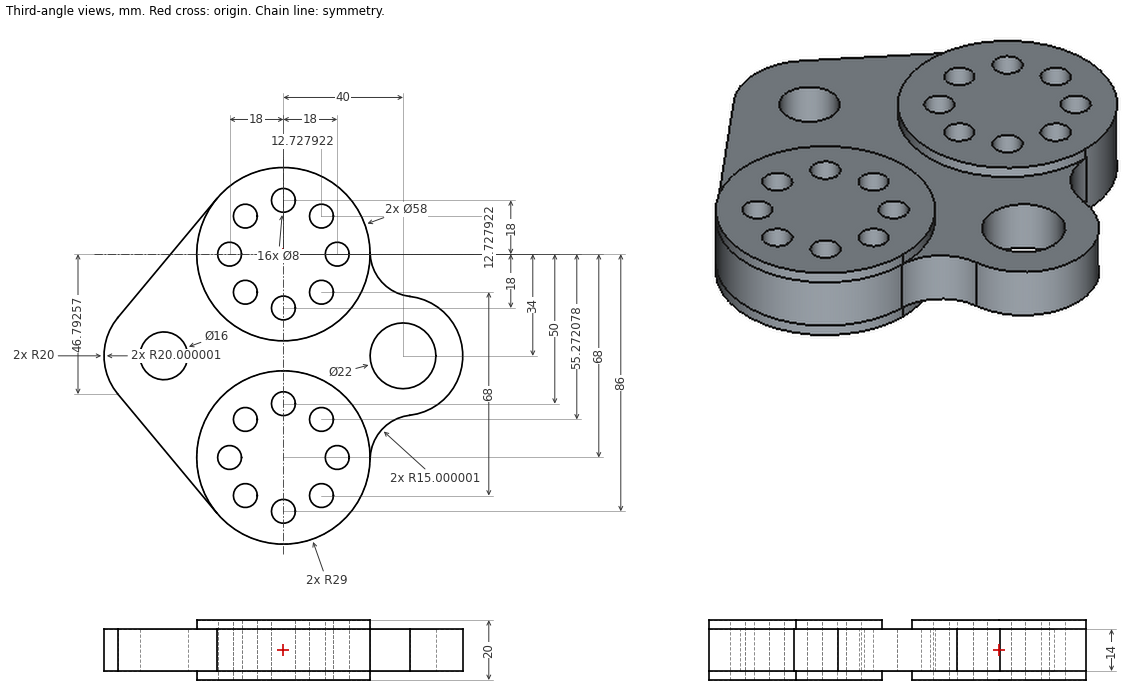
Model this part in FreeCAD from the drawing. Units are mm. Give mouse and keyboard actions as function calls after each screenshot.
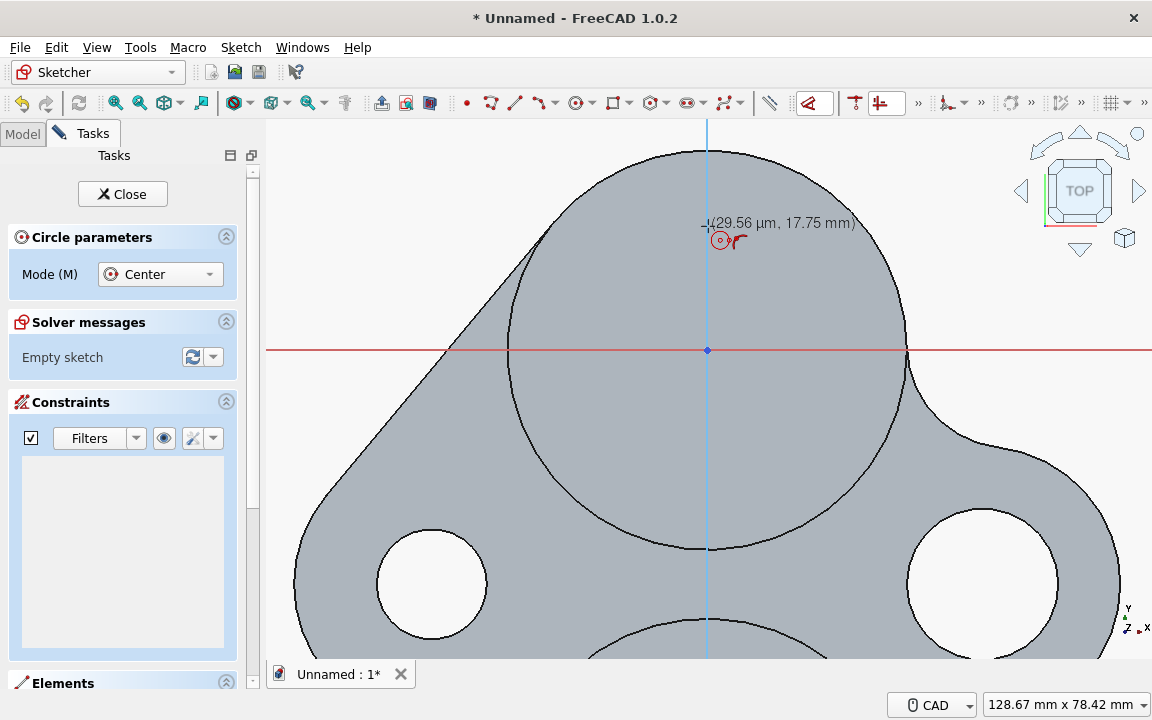
click(707, 226)
move(727, 207)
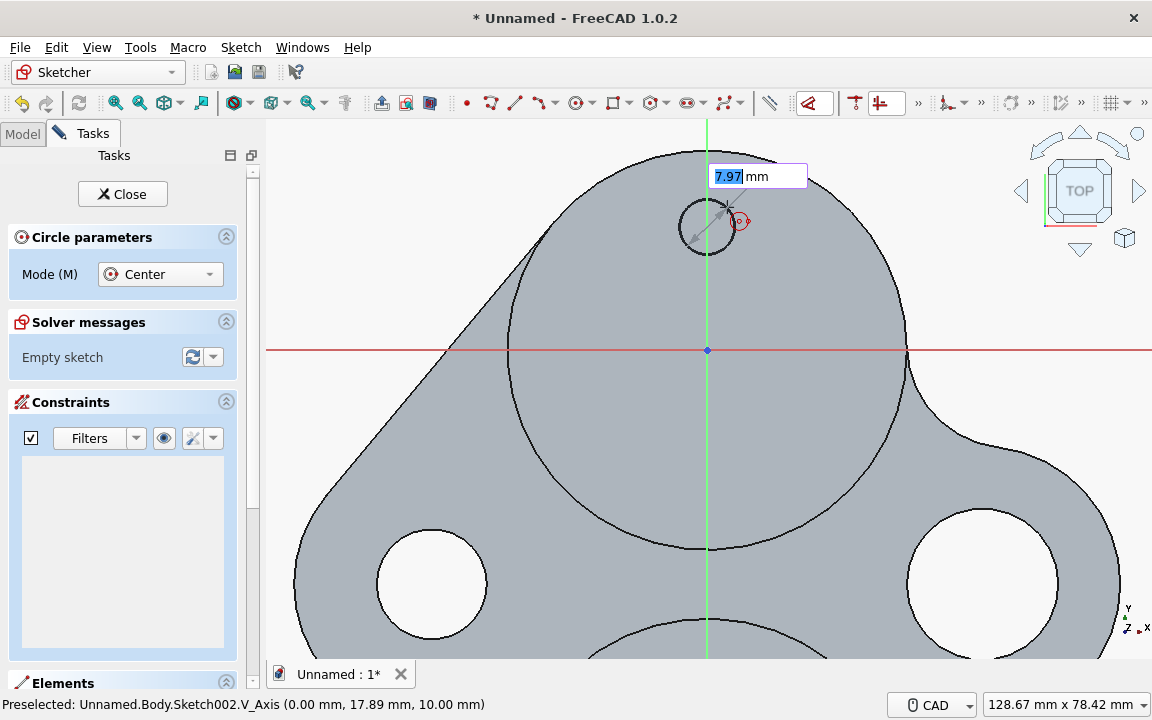
text(8)
key(Return)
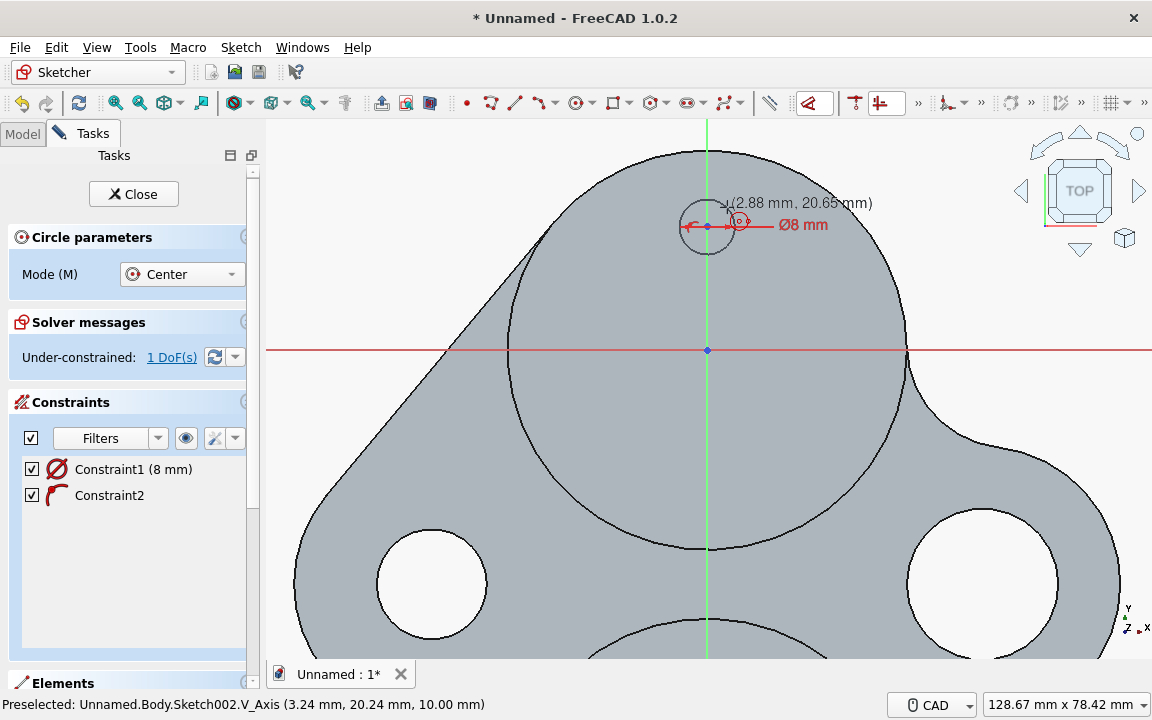
click(795, 263)
move(814, 243)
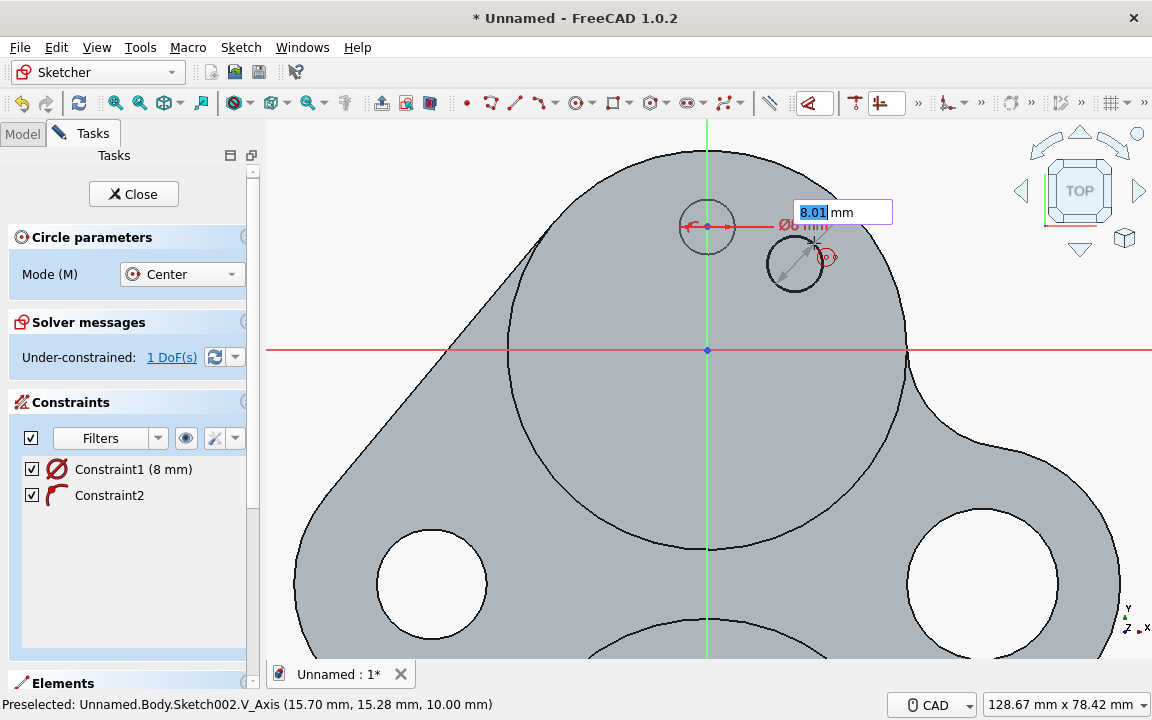
text(8)
key(Return)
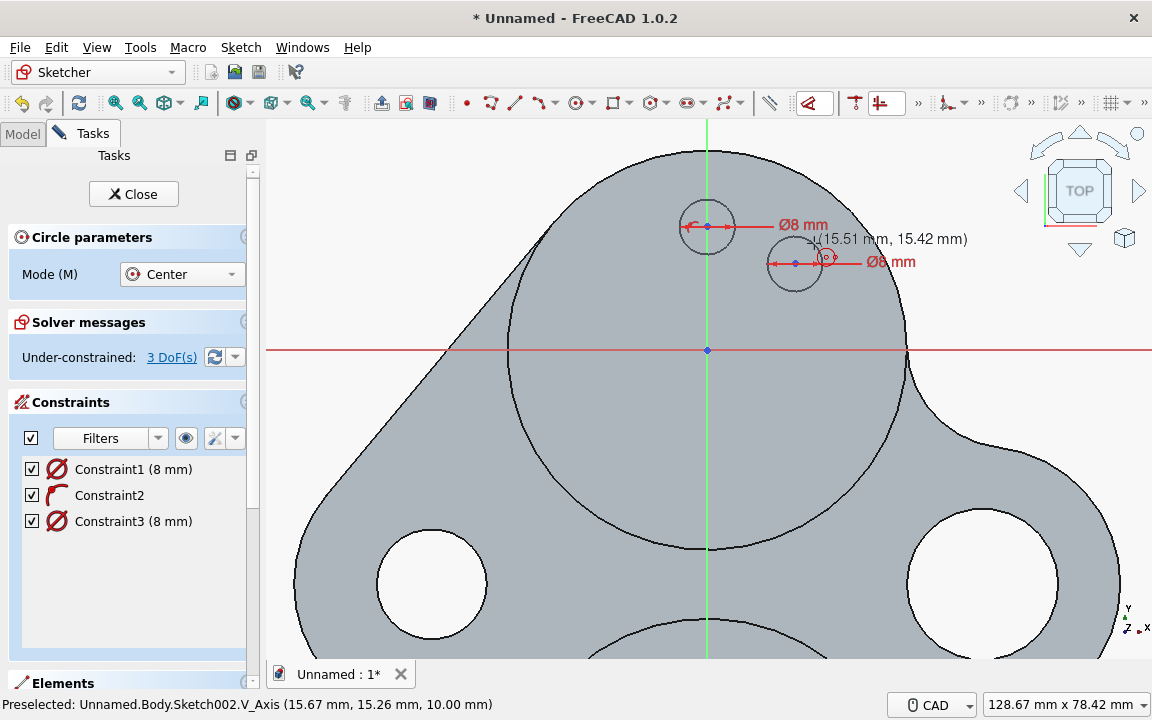
click(831, 350)
move(851, 331)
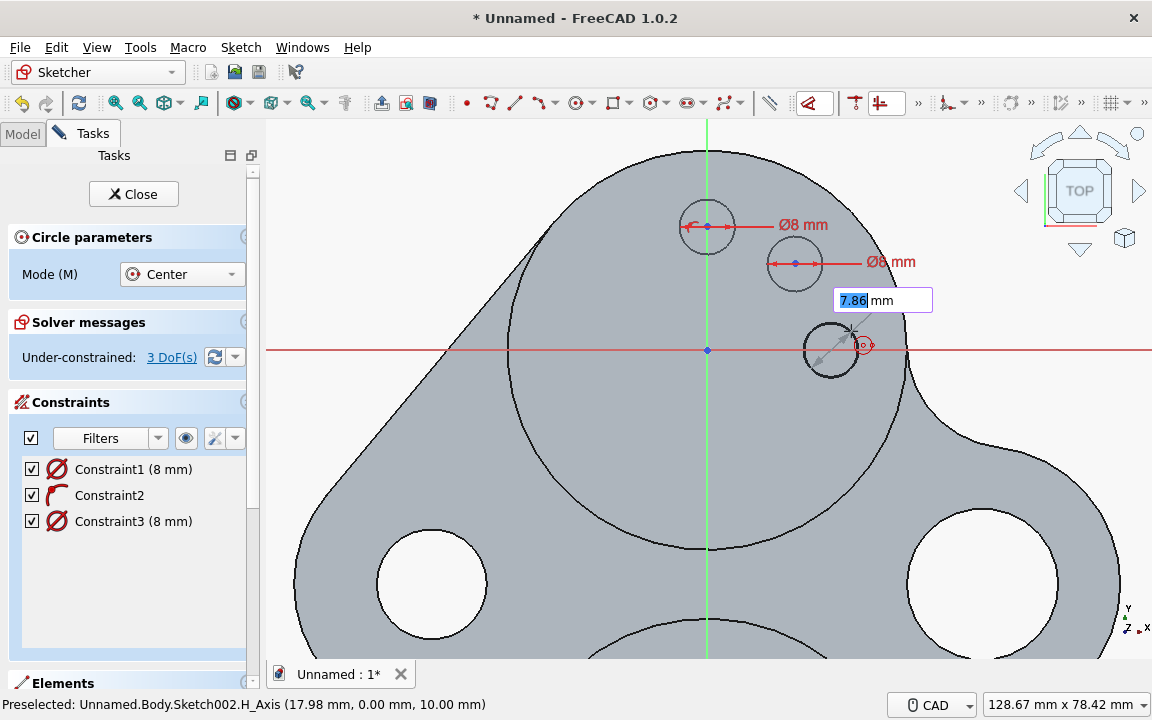
text(8)
key(Return)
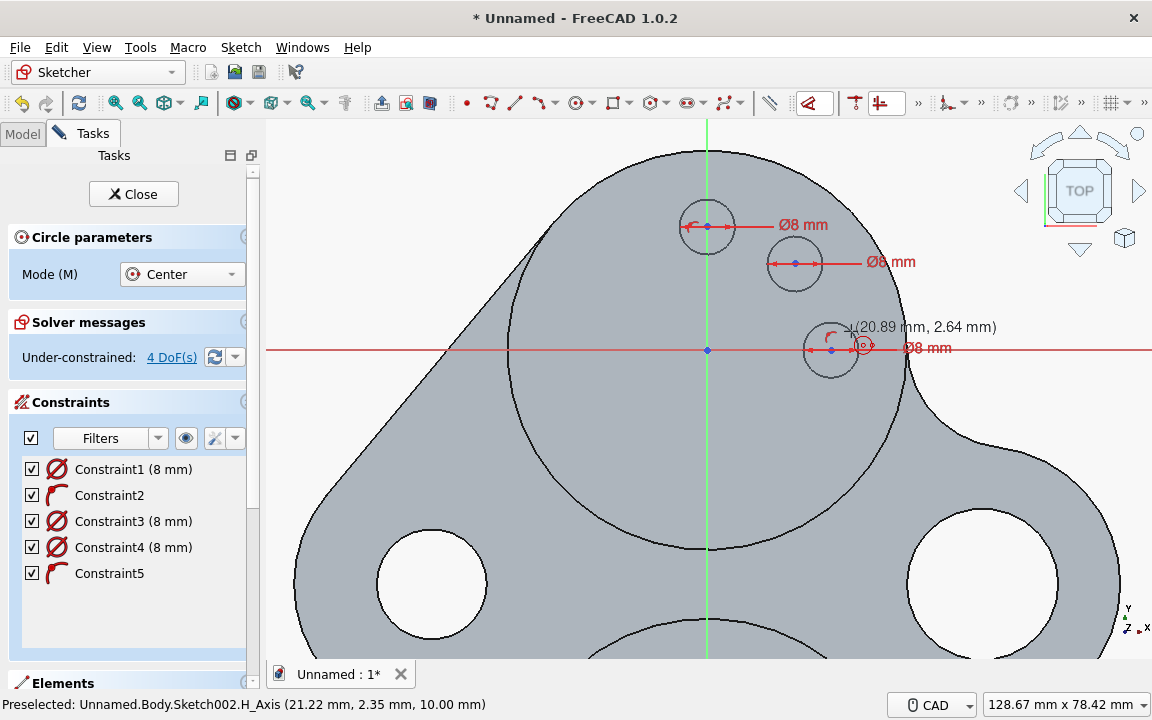
click(795, 438)
move(814, 418)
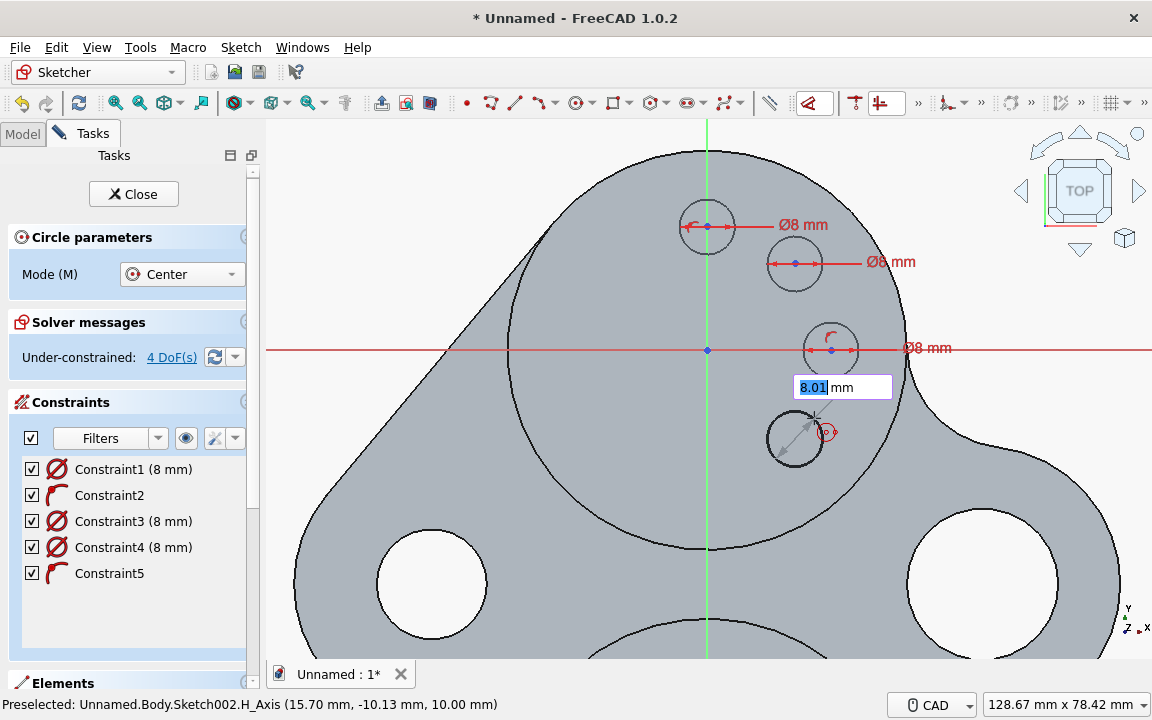
text(8)
key(Return)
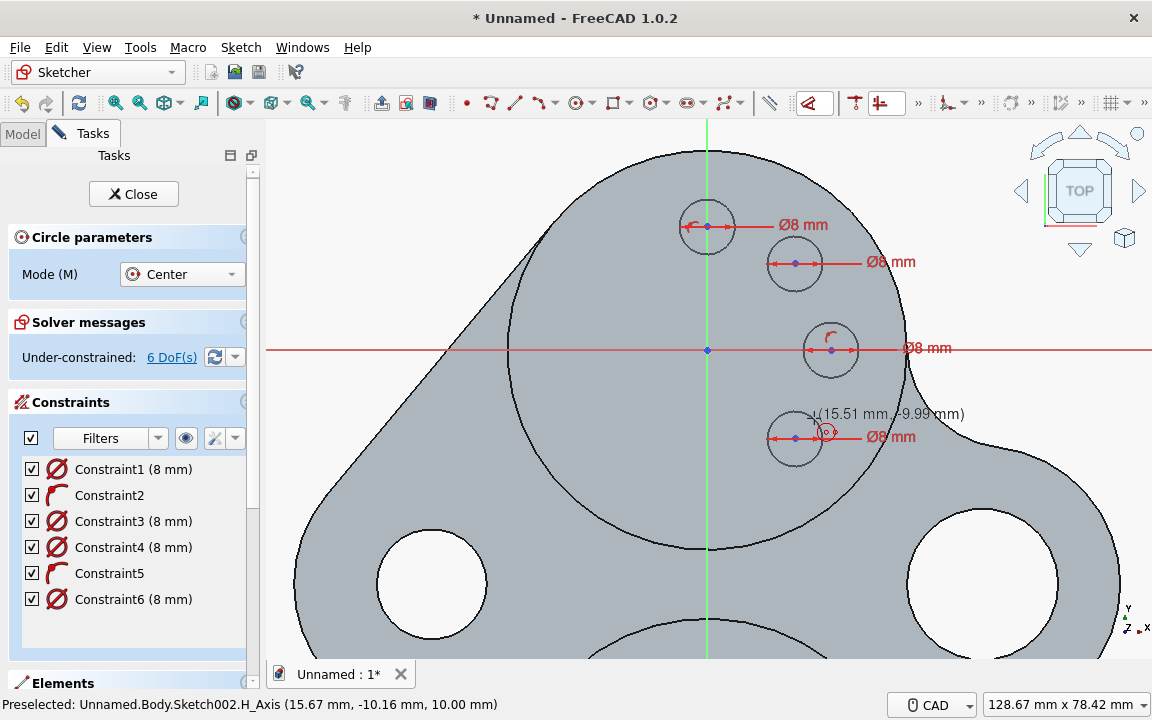
click(707, 474)
move(727, 455)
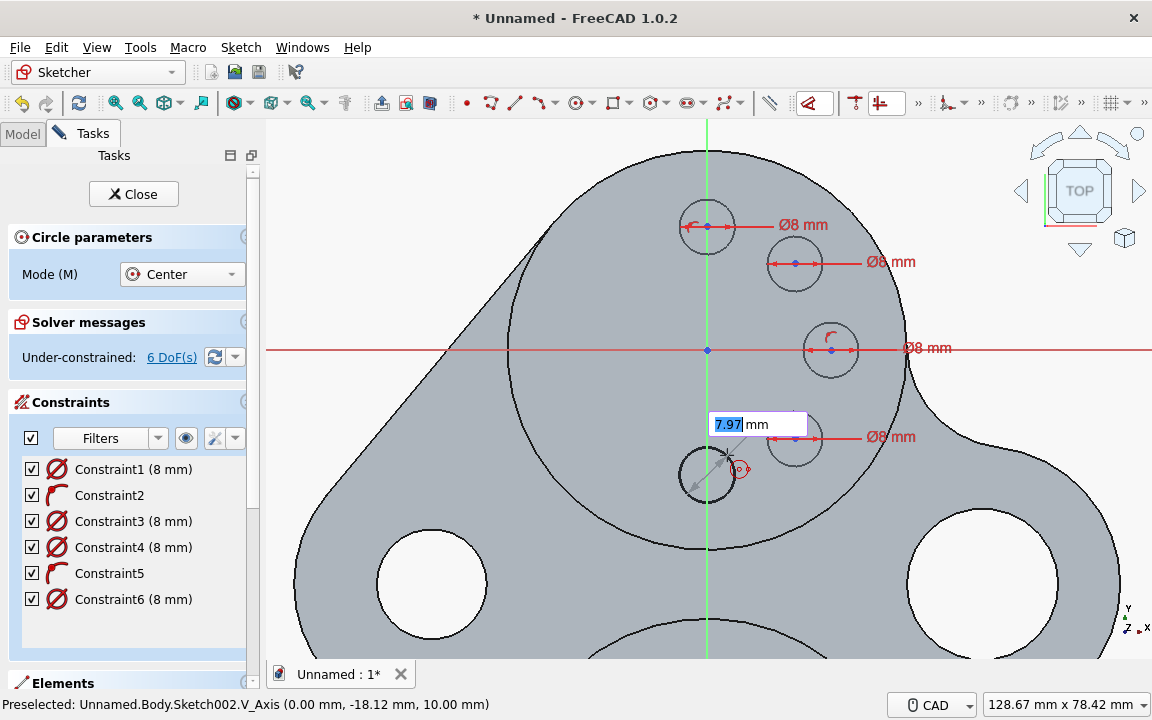
text(8)
key(Return)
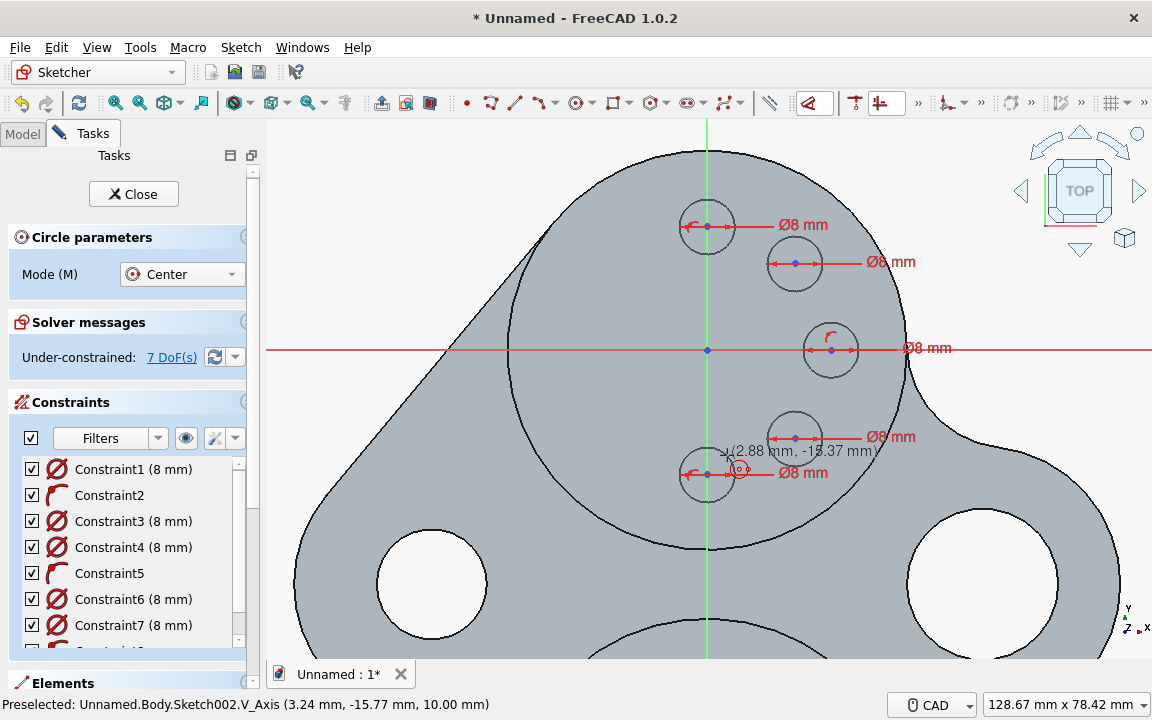
click(620, 438)
move(639, 418)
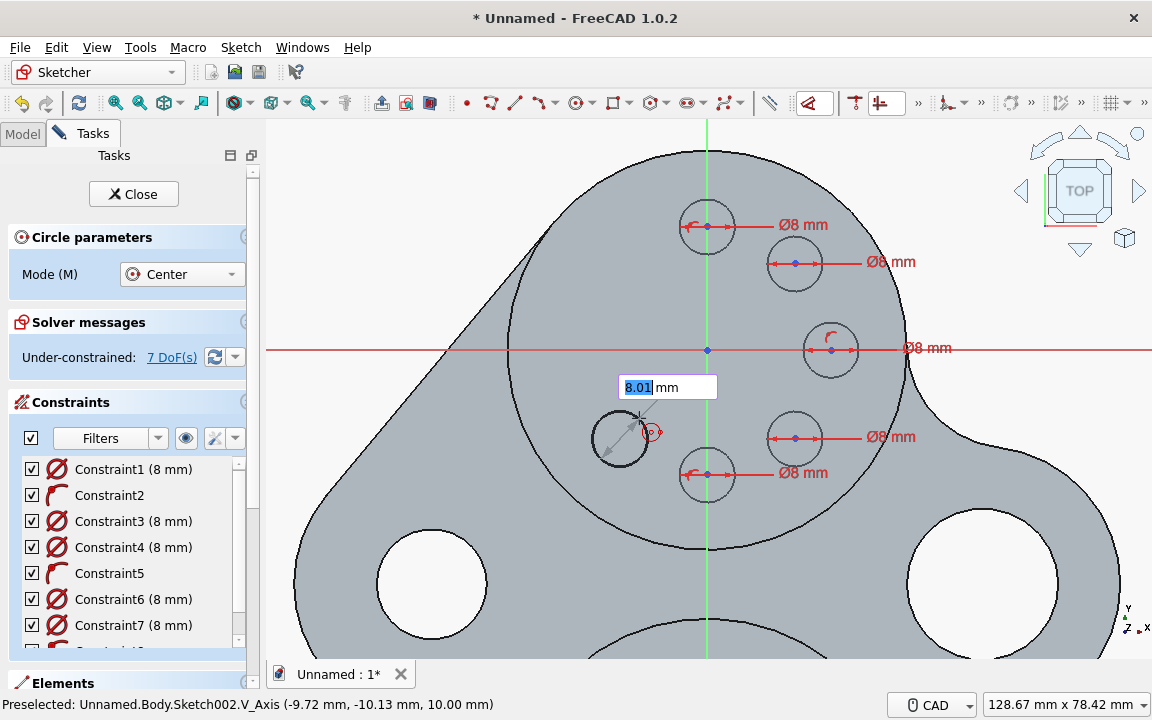
text(8)
key(Return)